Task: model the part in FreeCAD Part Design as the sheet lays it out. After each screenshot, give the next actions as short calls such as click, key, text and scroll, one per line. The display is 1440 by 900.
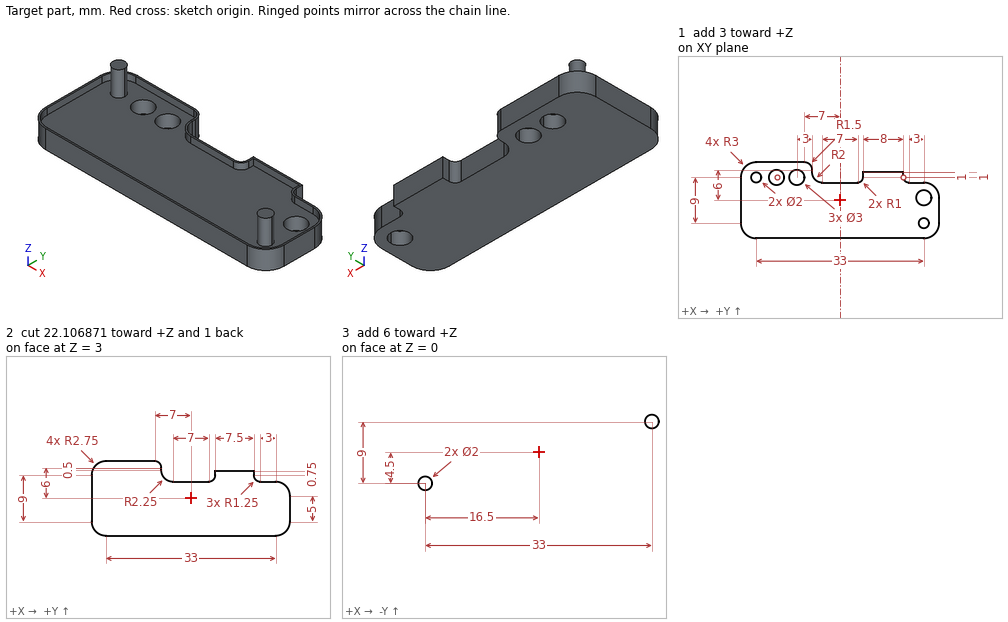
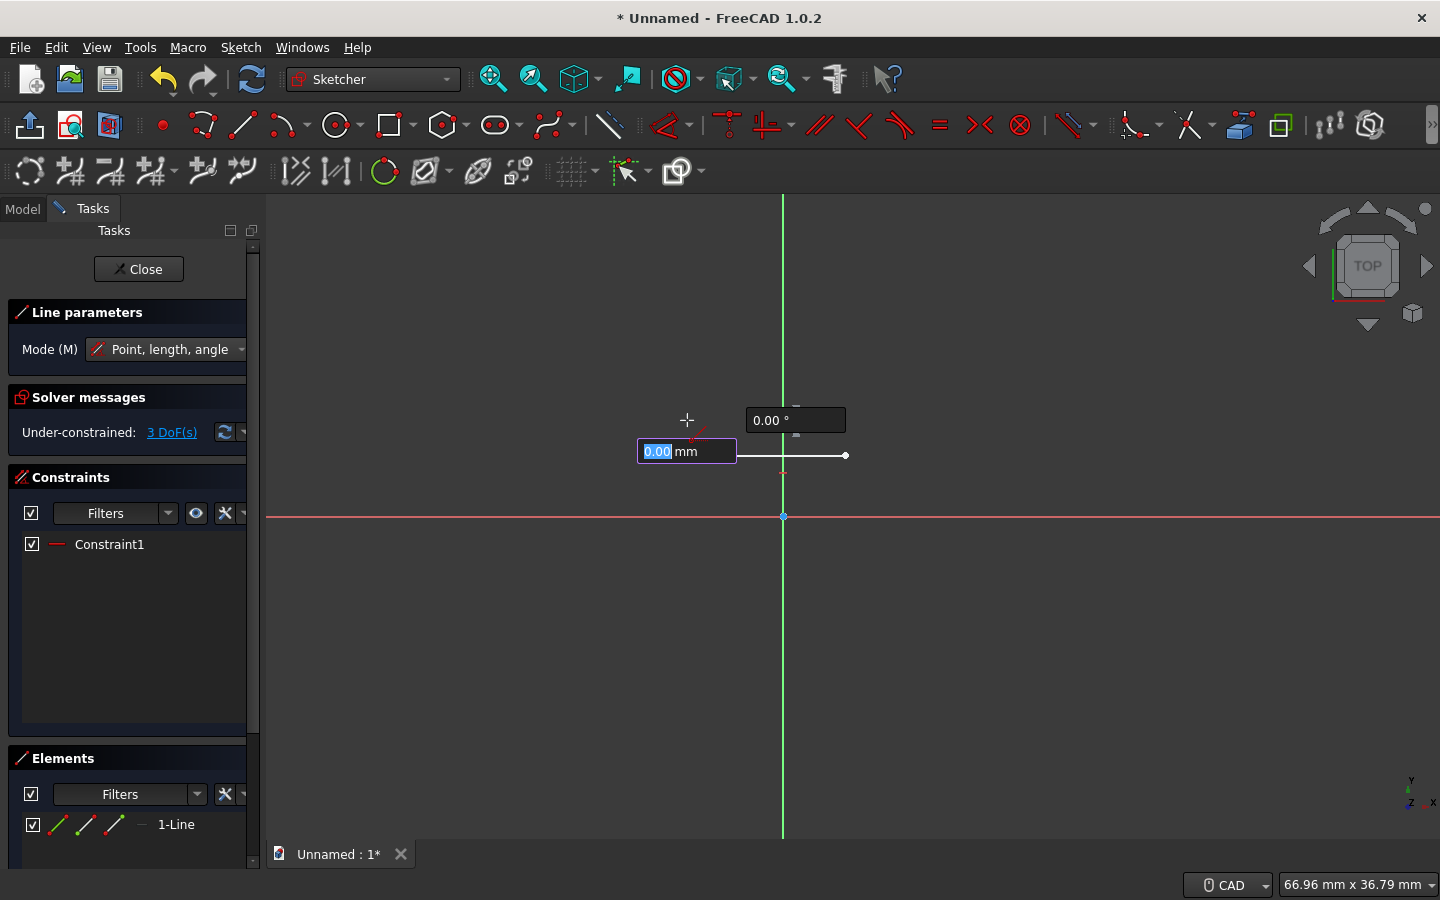
scroll(687, 411, up, 3)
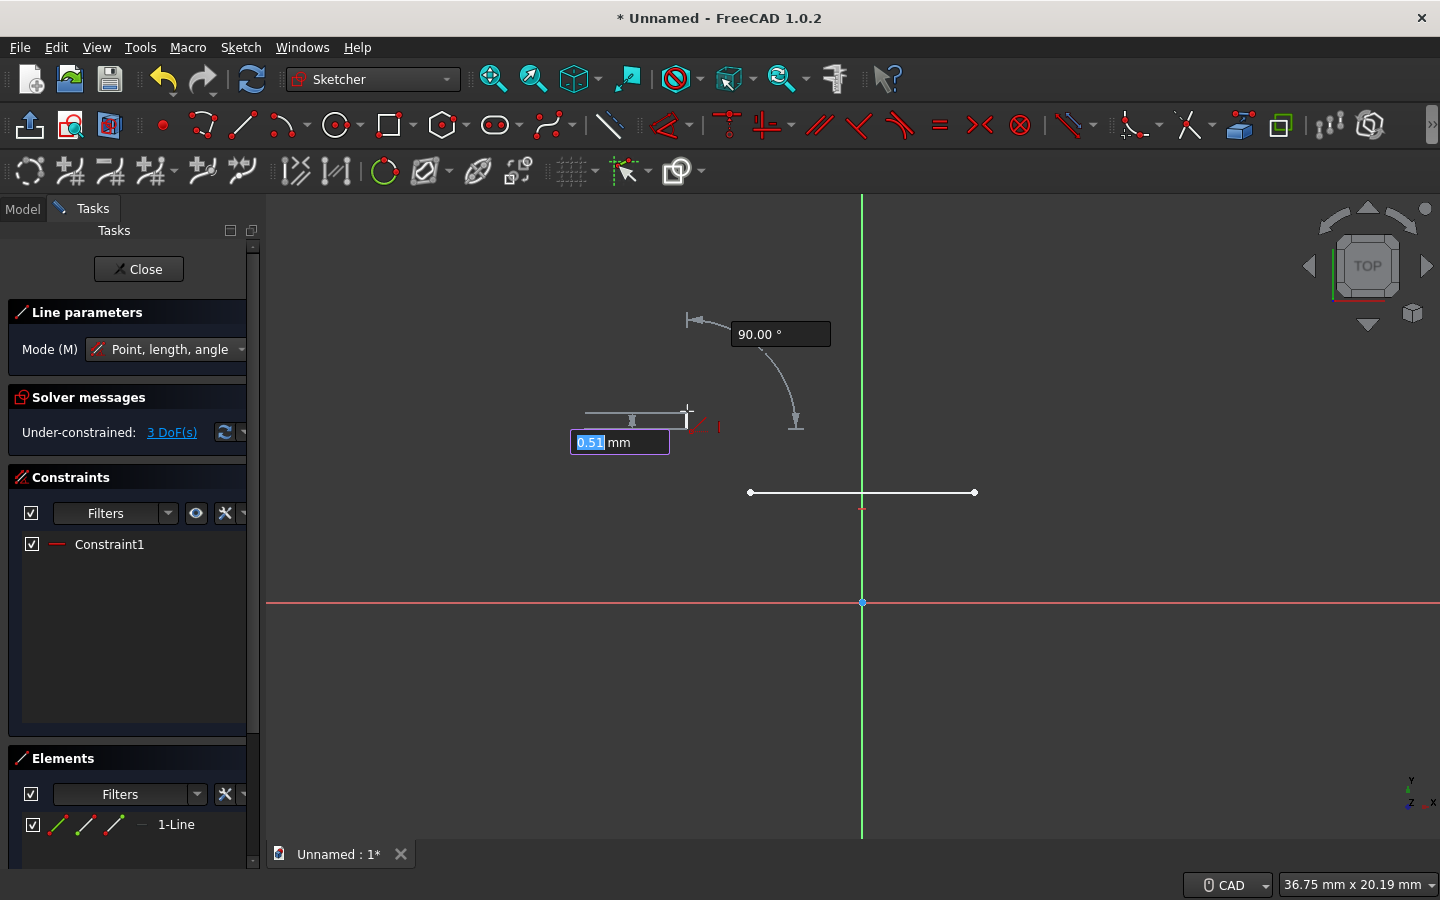
click(687, 411)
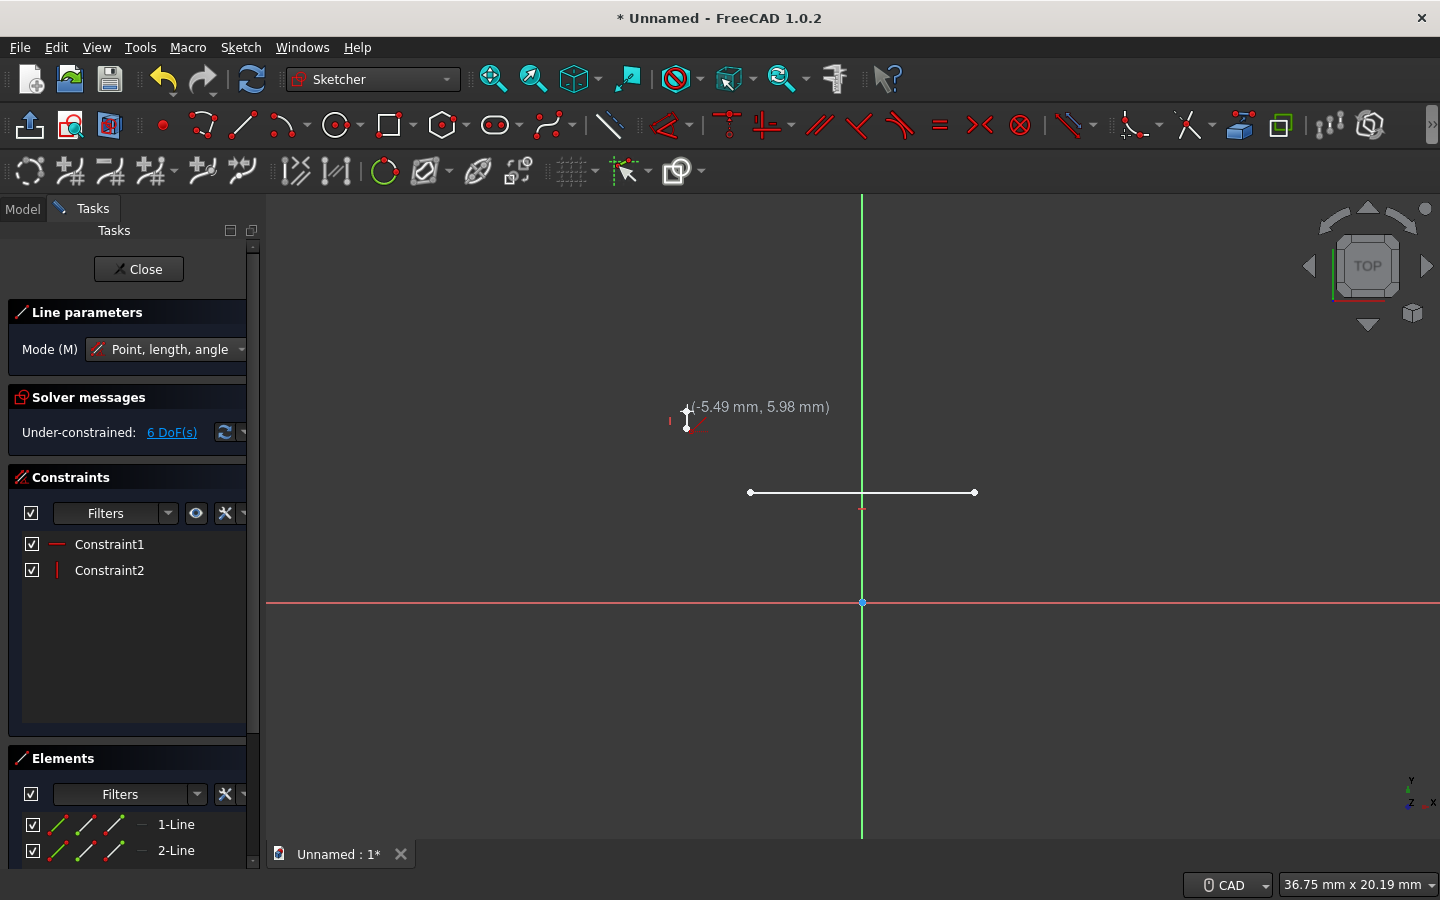
click(639, 363)
click(335, 363)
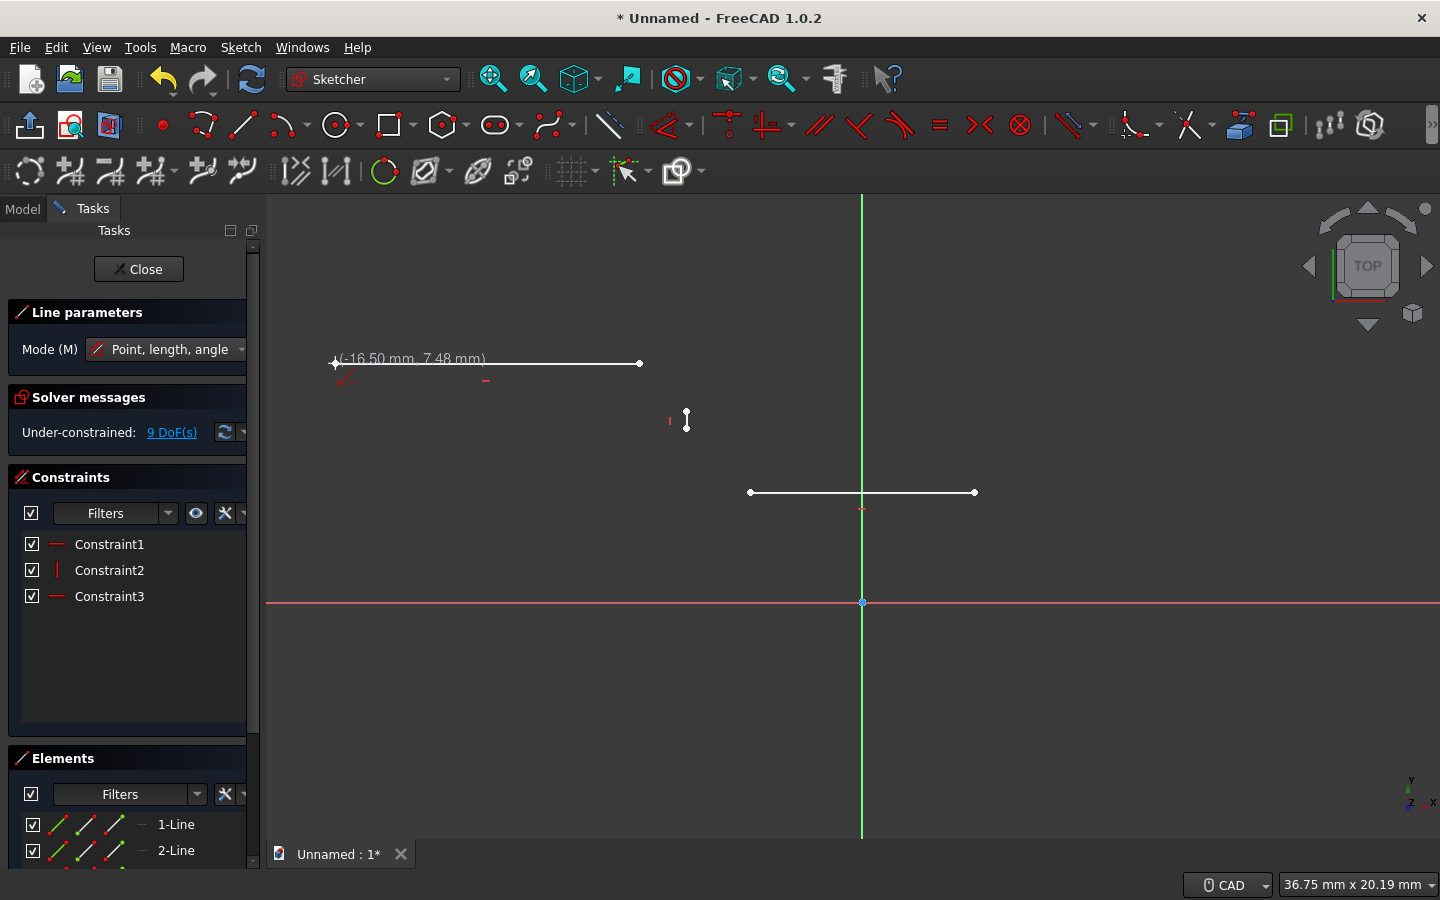
scroll(690, 411, down, 3)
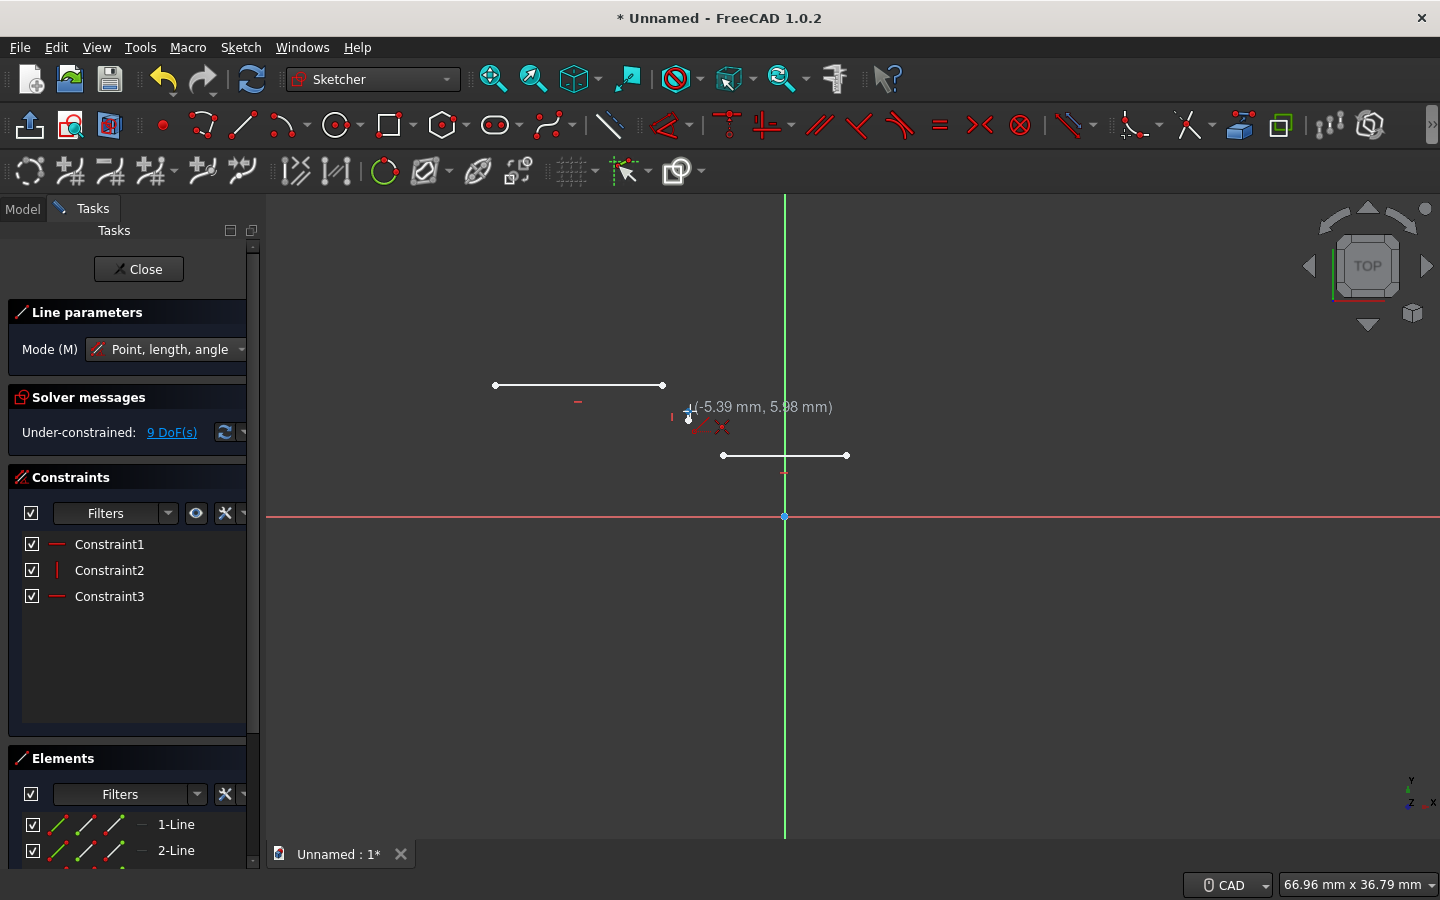
click(443, 438)
click(443, 595)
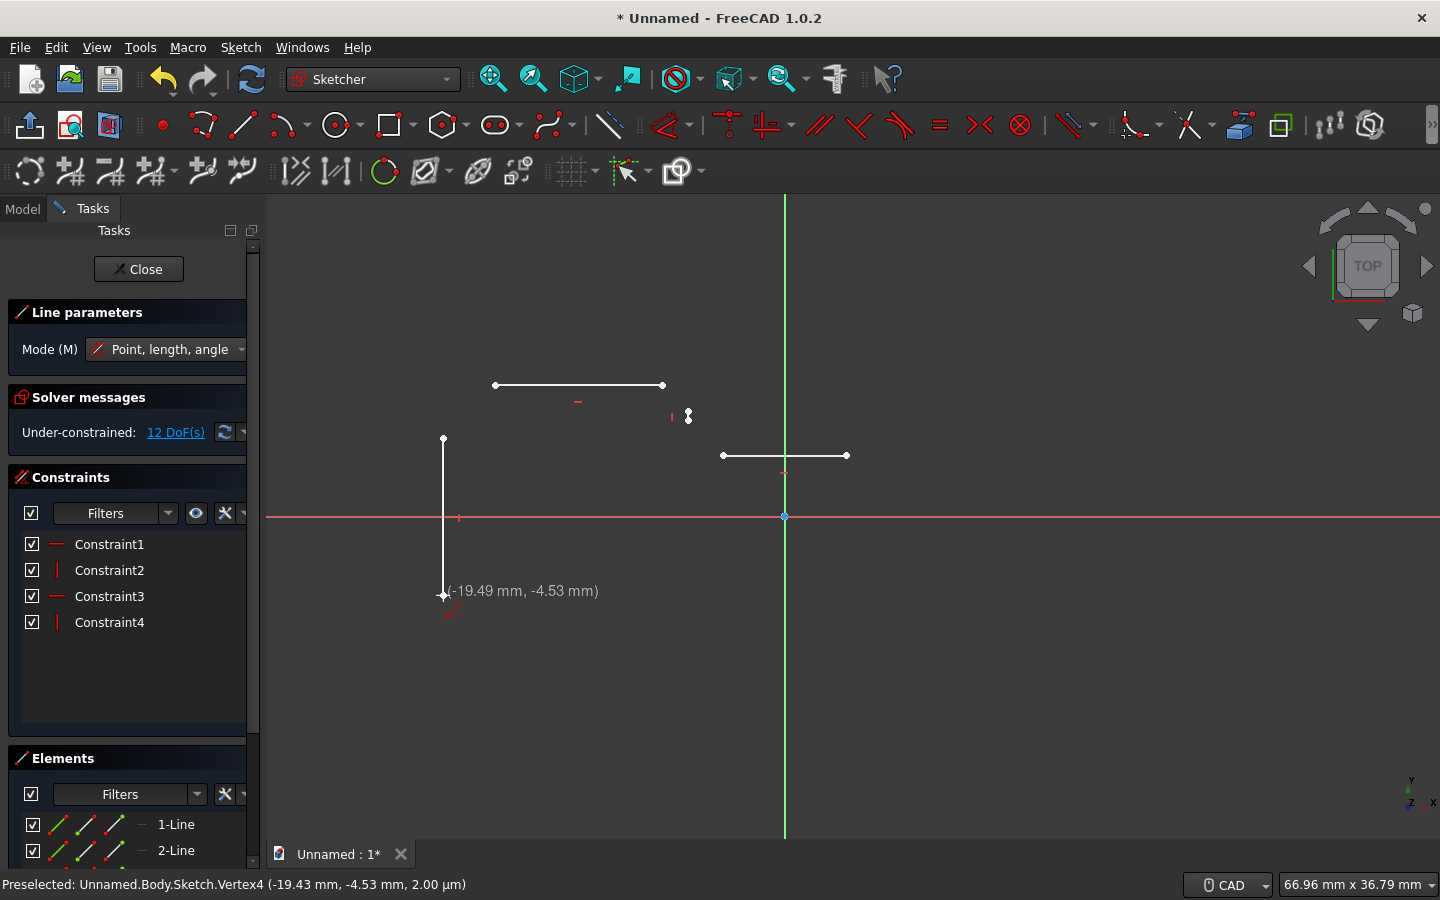
click(495, 648)
click(1074, 648)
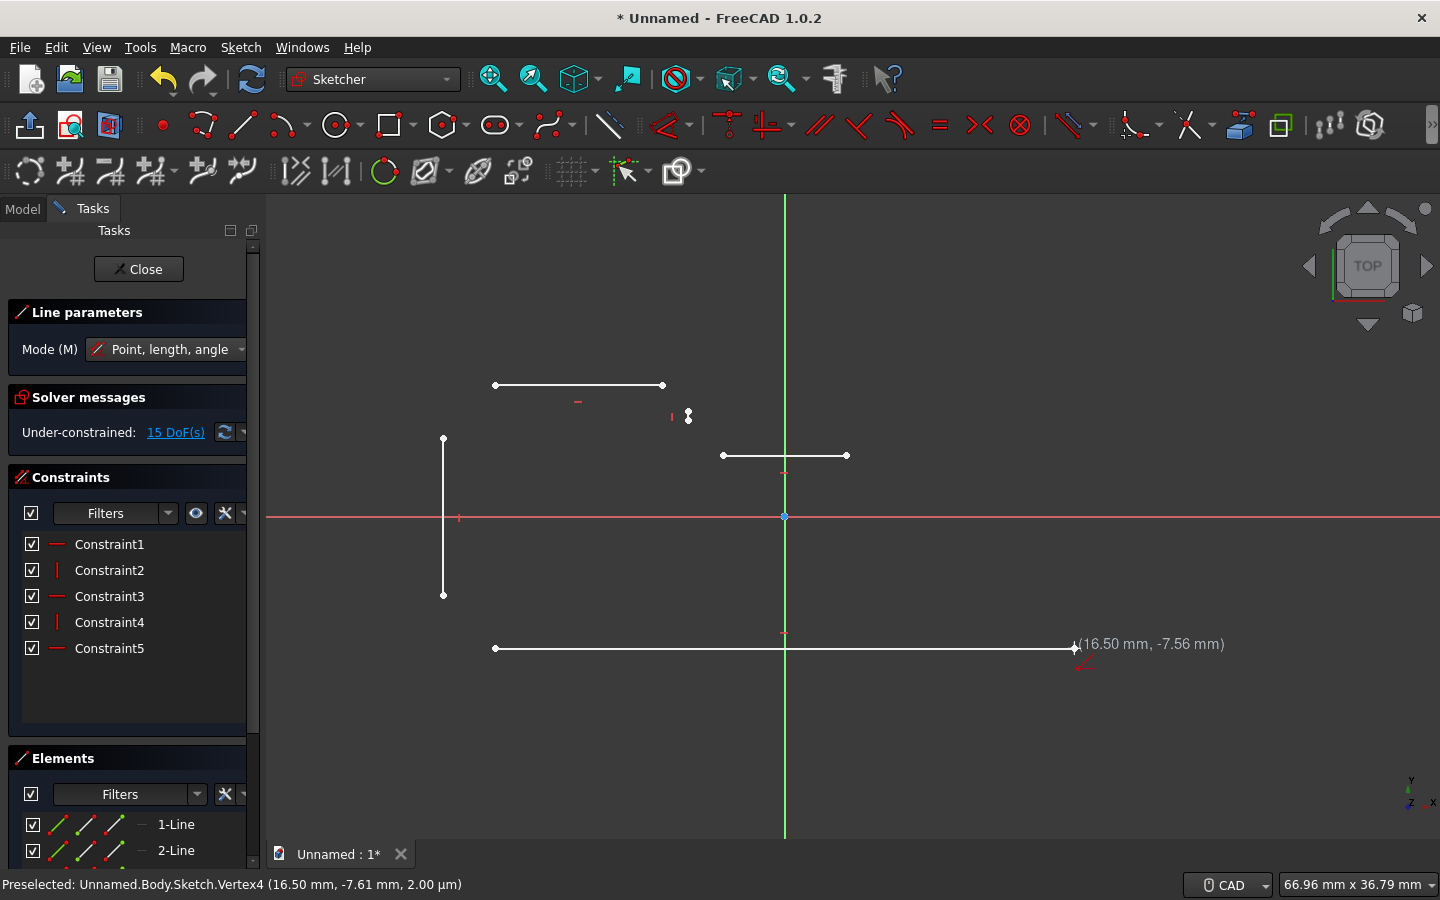
click(1127, 595)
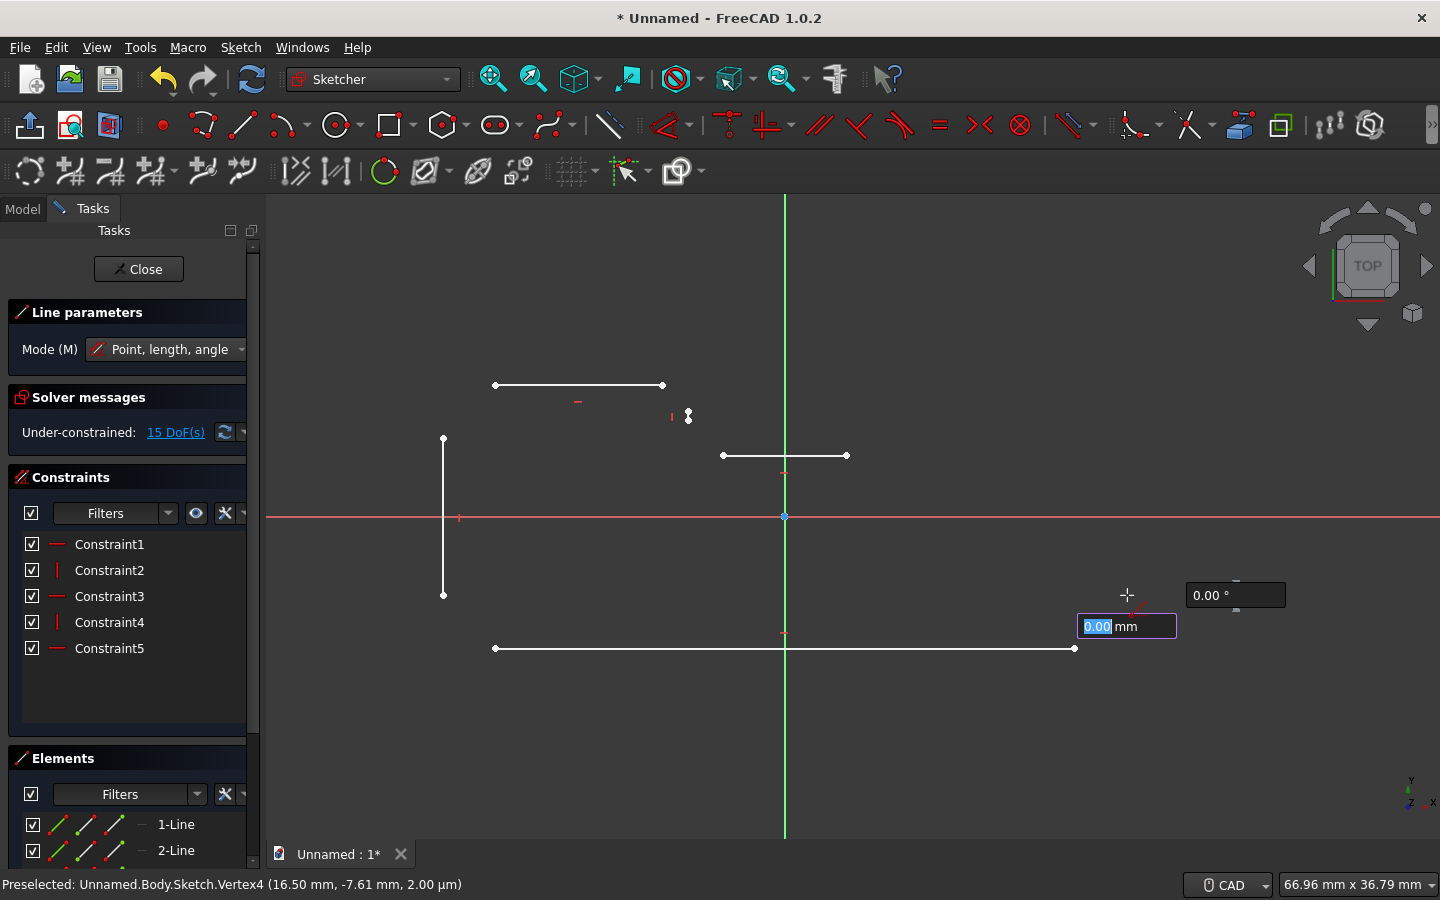
scroll(1127, 508, up, 3)